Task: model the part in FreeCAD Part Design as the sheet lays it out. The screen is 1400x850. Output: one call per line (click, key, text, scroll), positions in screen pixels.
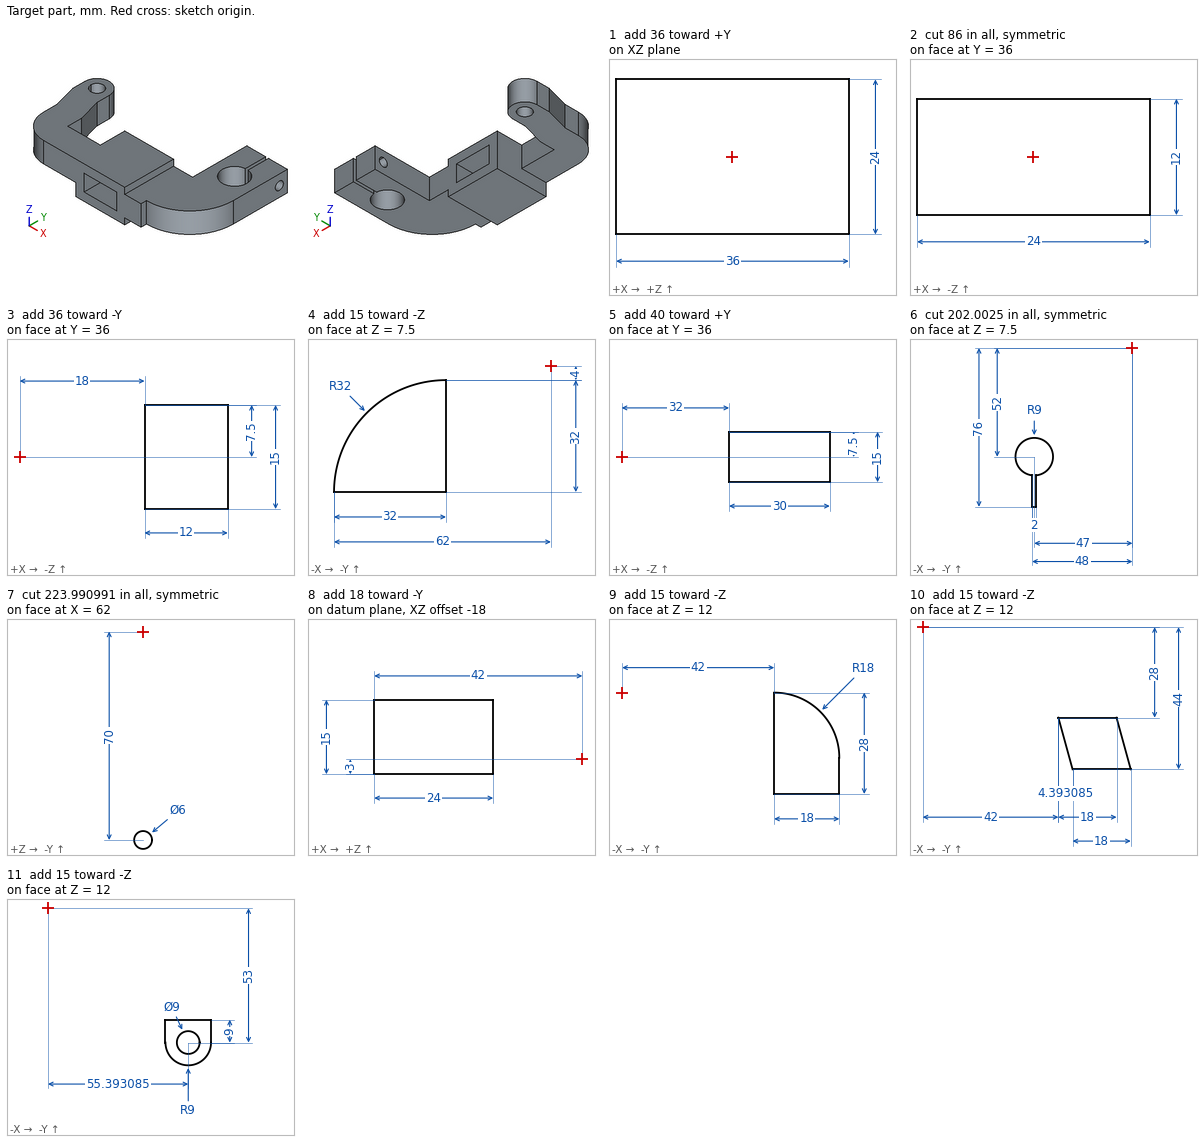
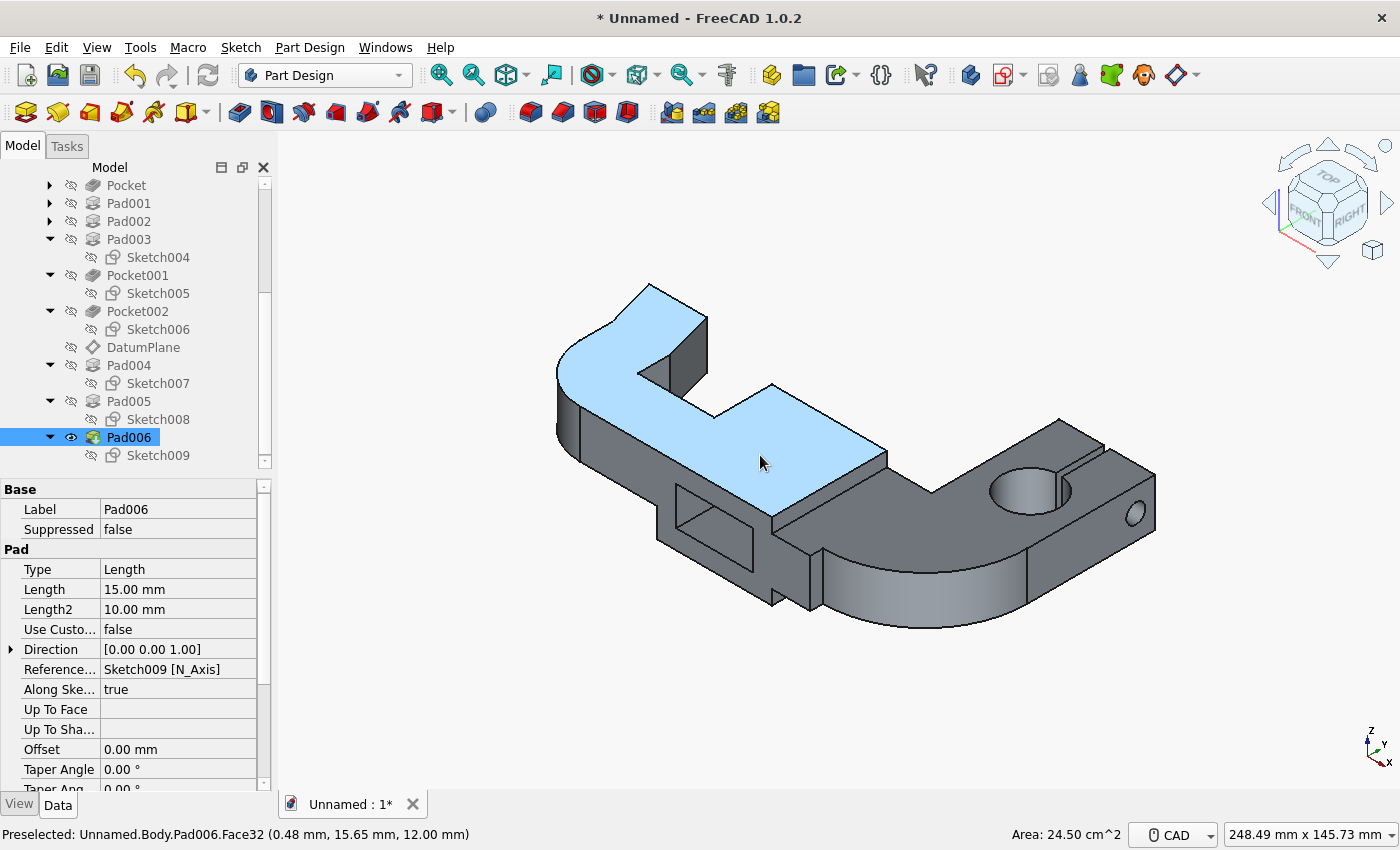
click(1004, 76)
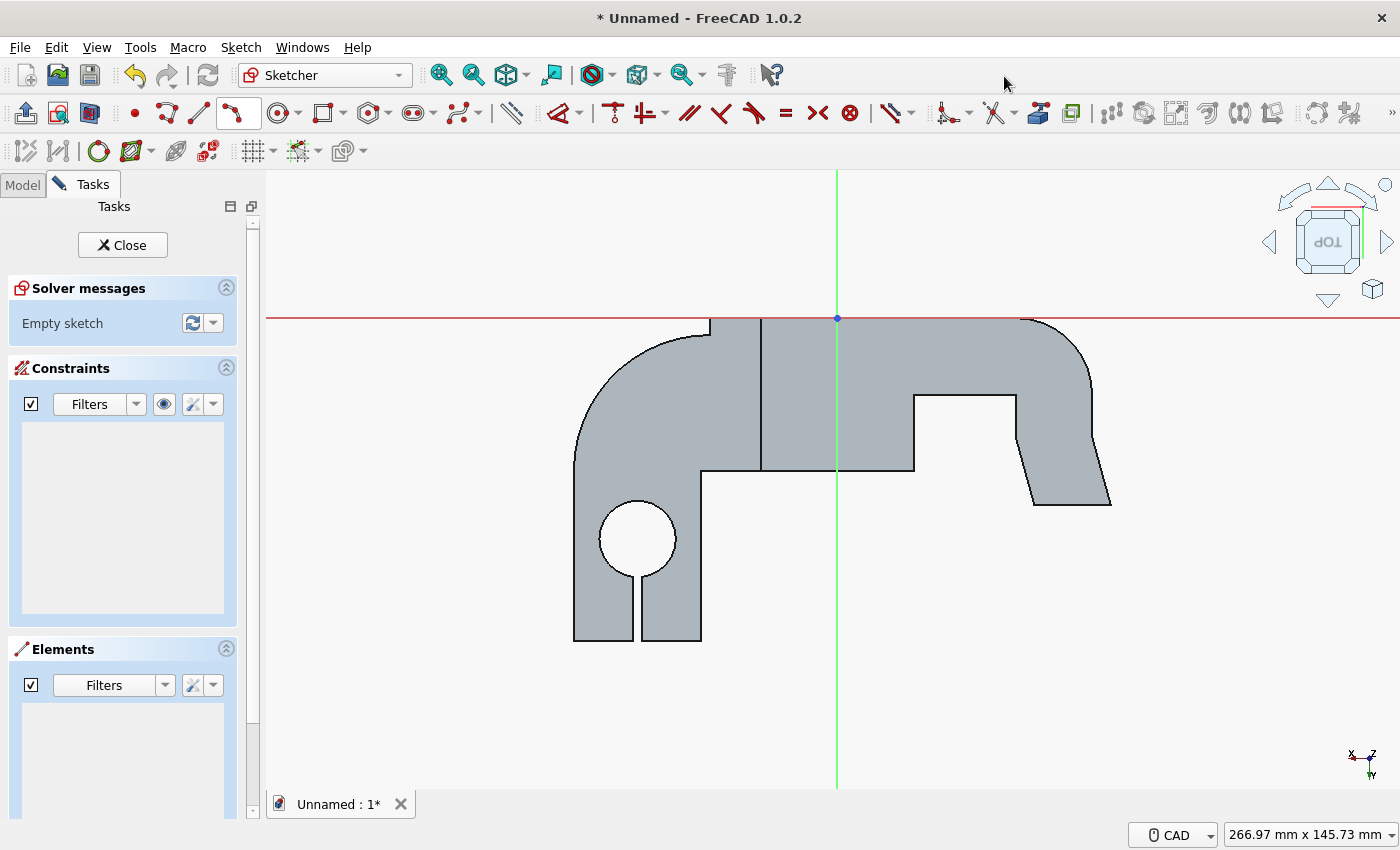
scroll(1150, 559, up, 8)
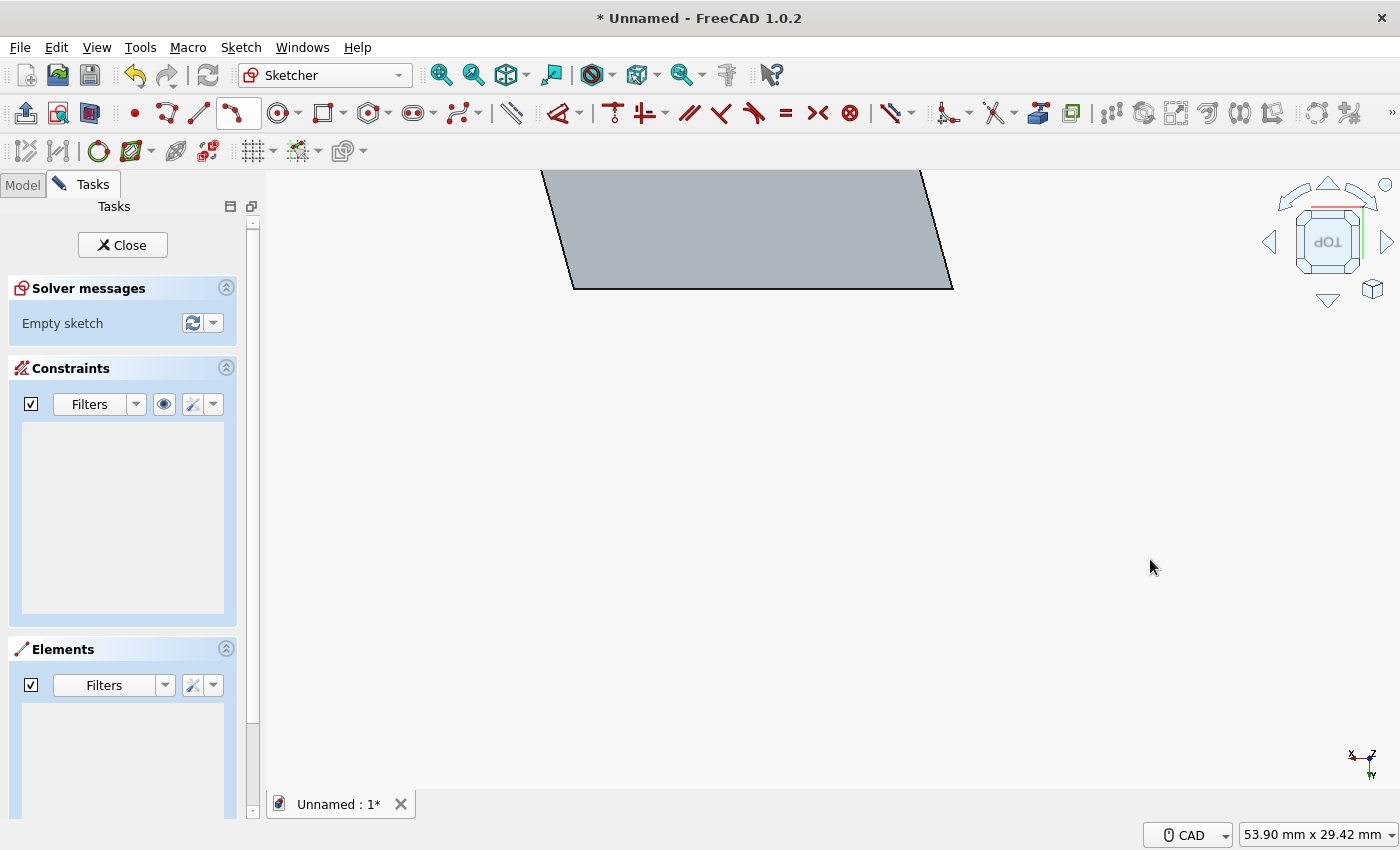
click(168, 114)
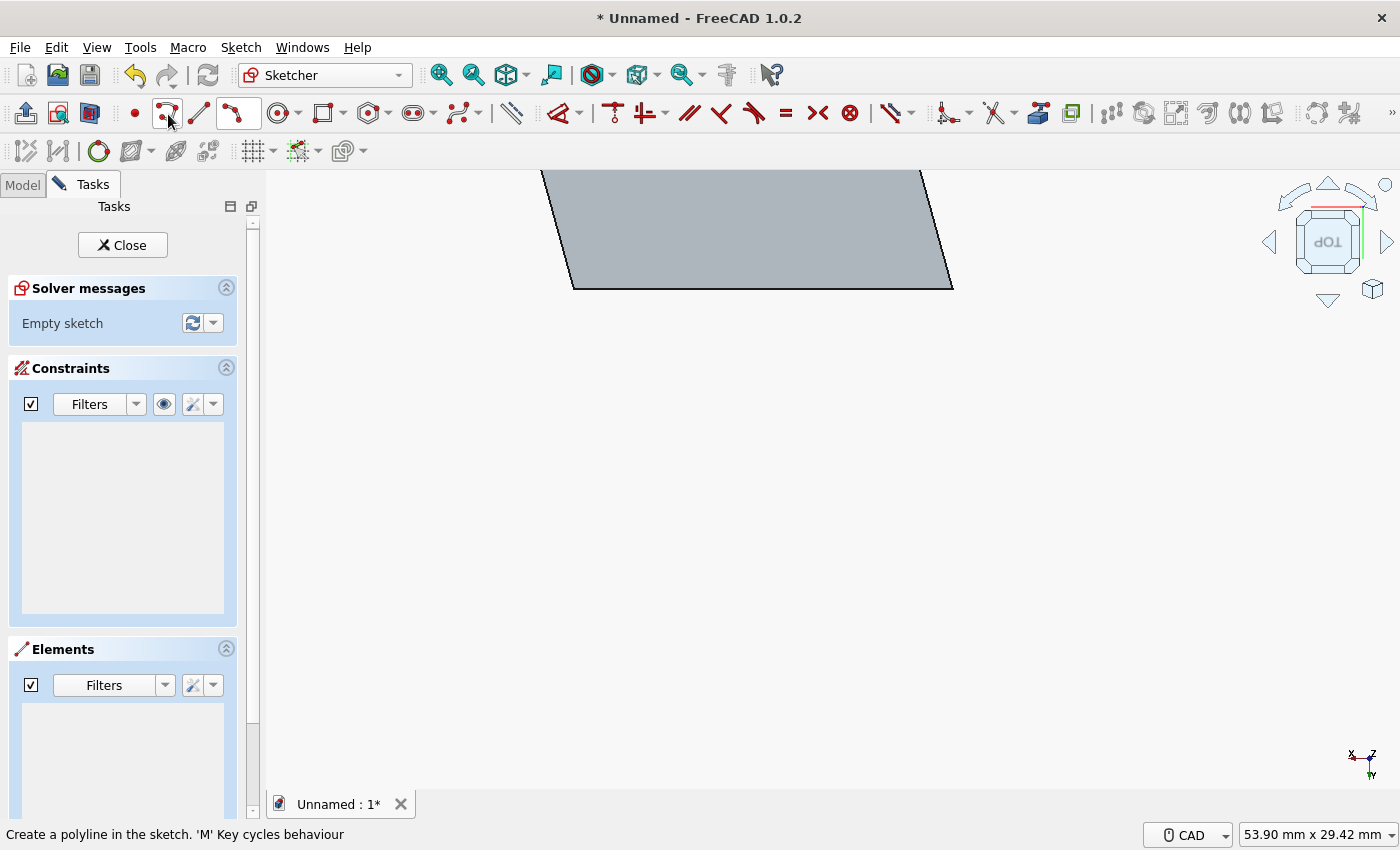
click(953, 478)
click(953, 289)
click(574, 289)
click(574, 478)
right_click(574, 478)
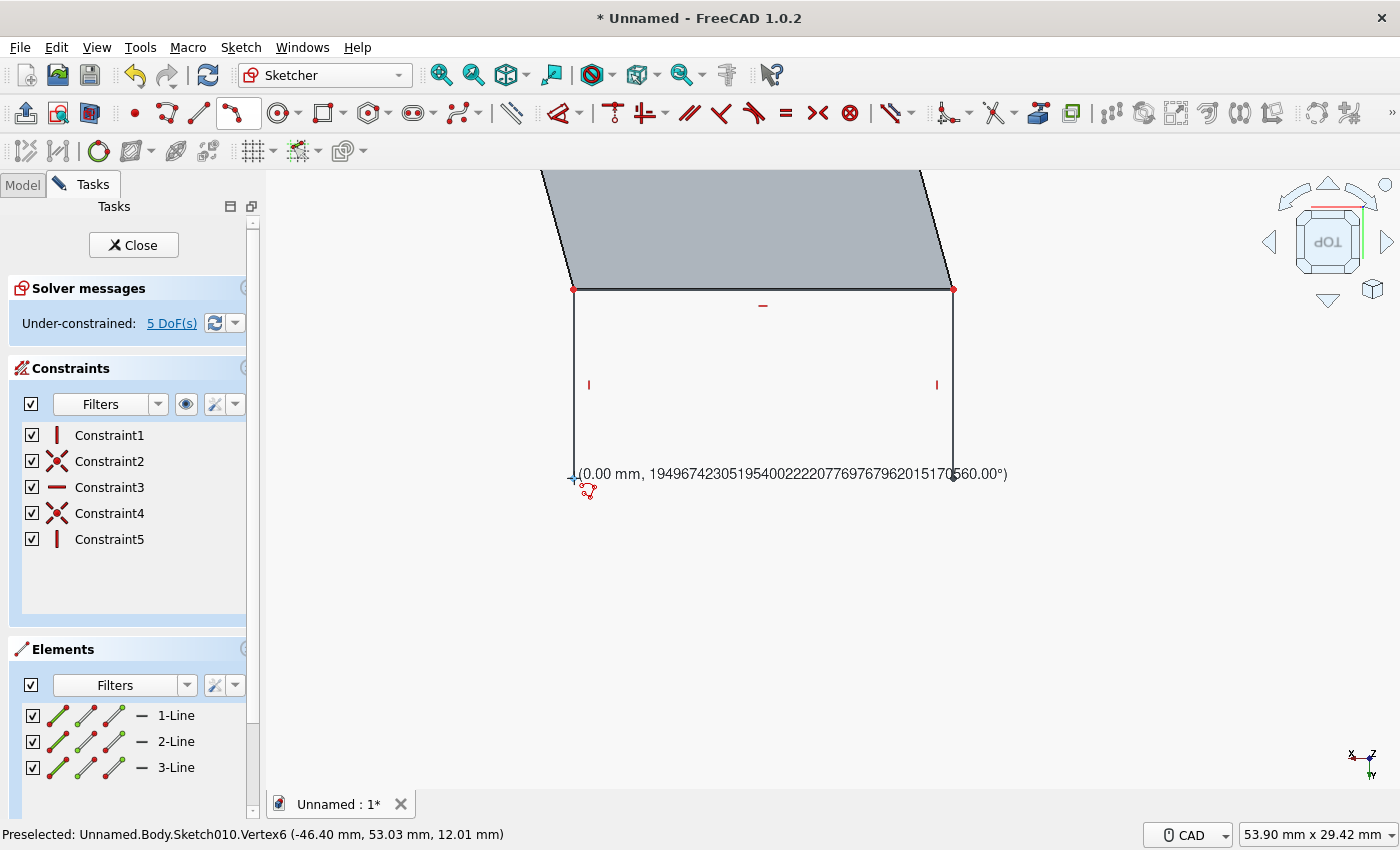
key(g)
key(3)
key(a)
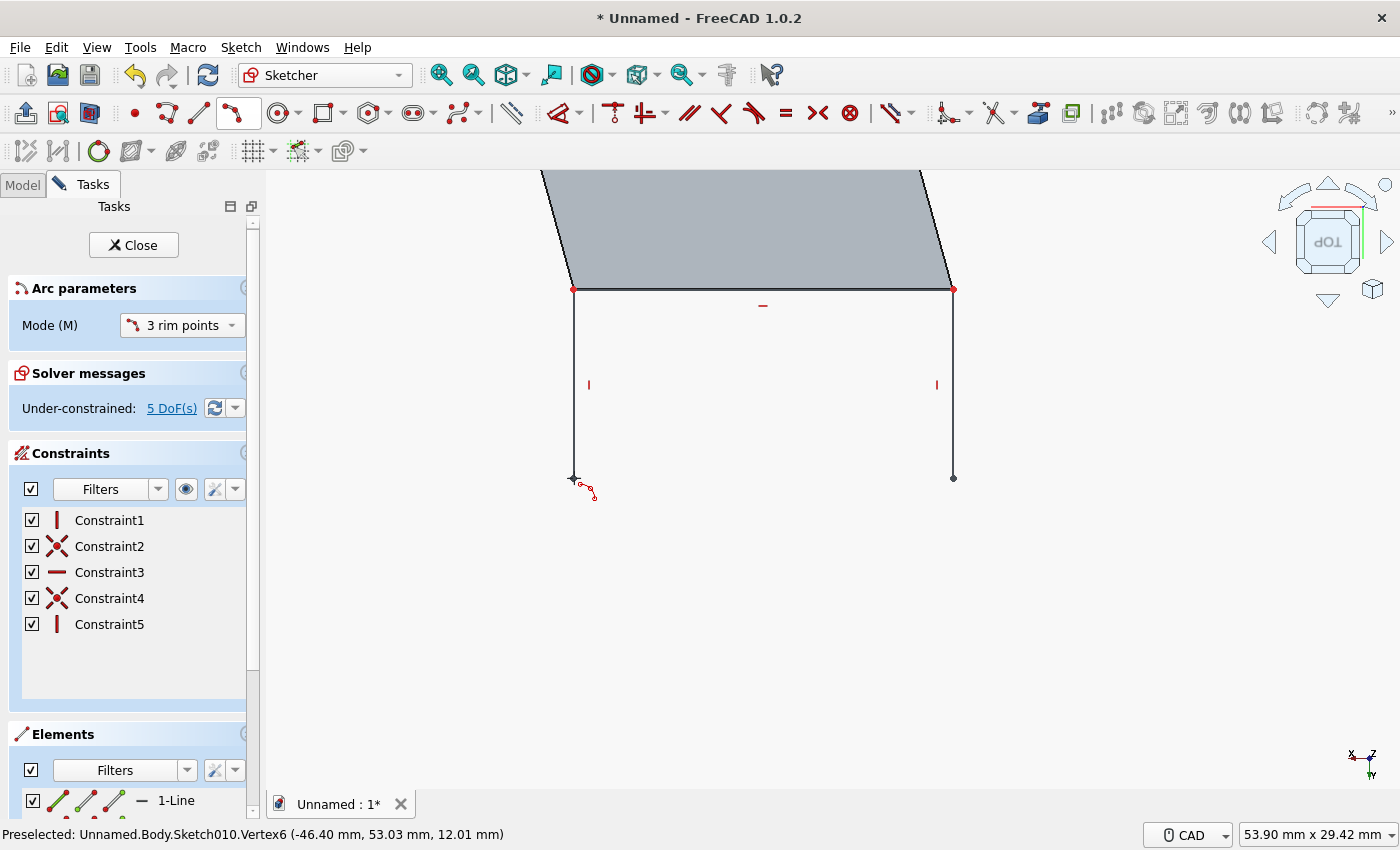
click(574, 479)
click(953, 479)
click(763, 668)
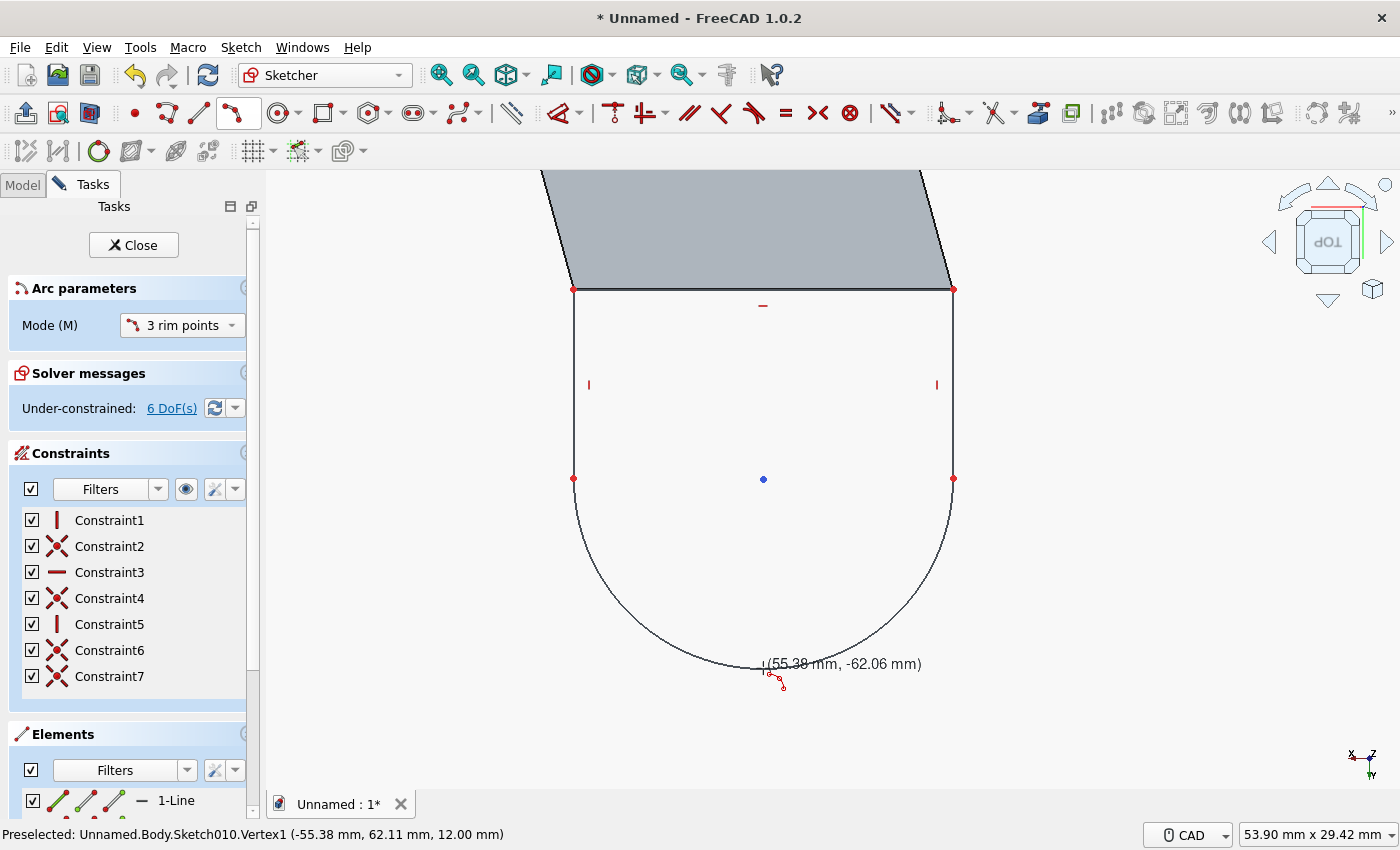
click(278, 114)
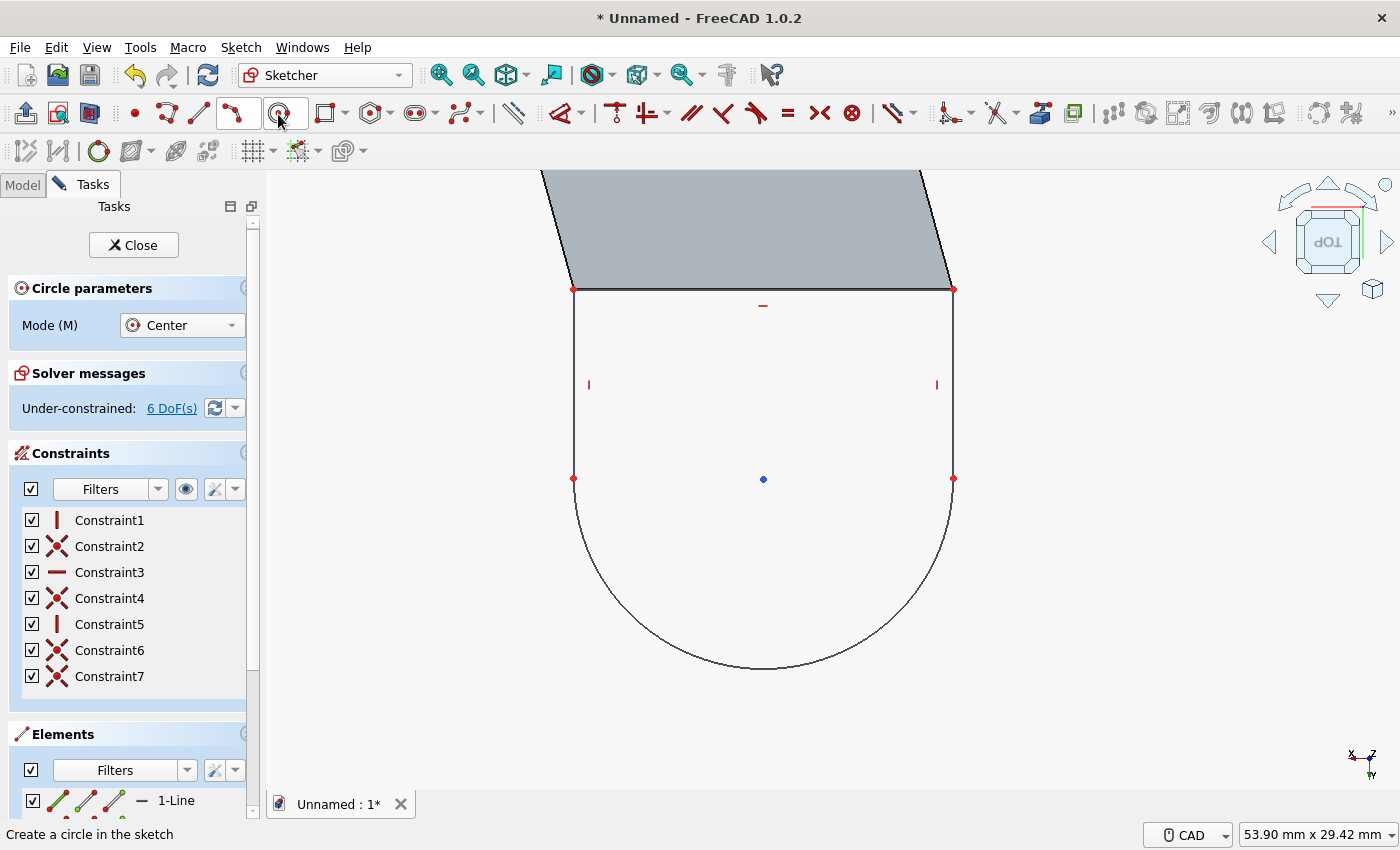
click(763, 478)
click(830, 411)
key(Escape)